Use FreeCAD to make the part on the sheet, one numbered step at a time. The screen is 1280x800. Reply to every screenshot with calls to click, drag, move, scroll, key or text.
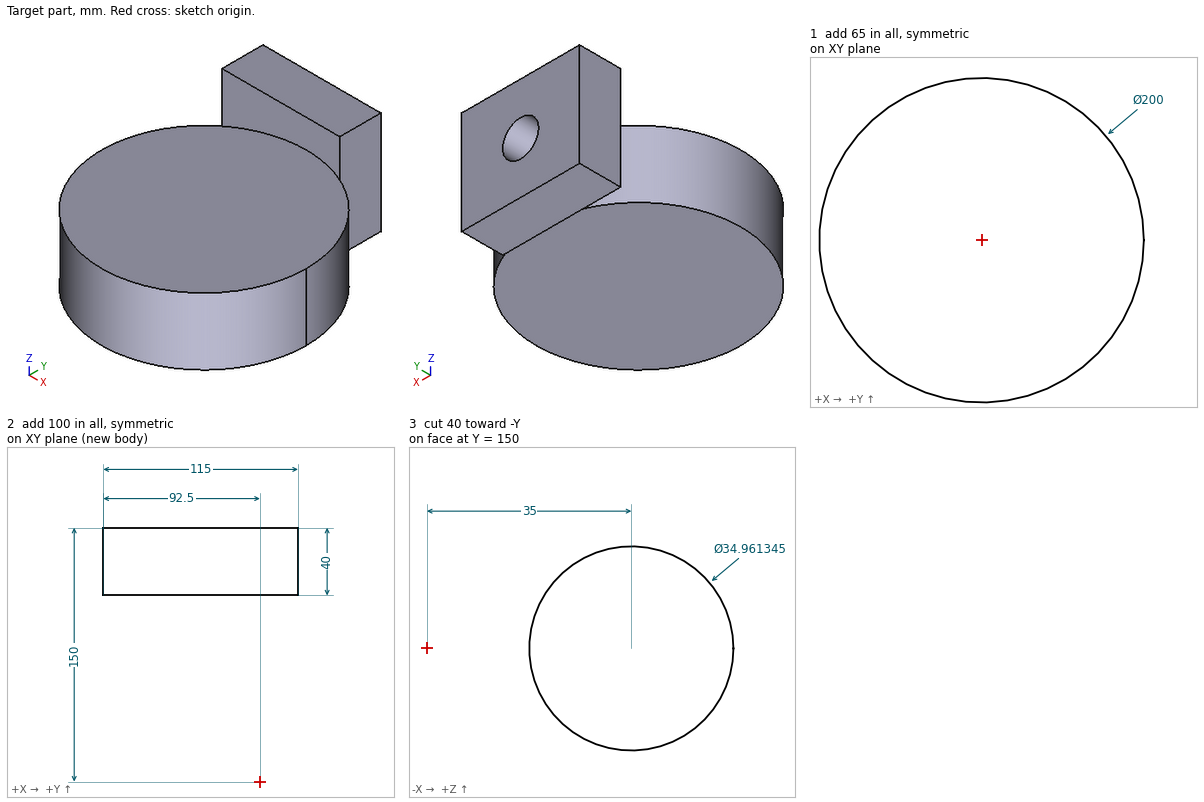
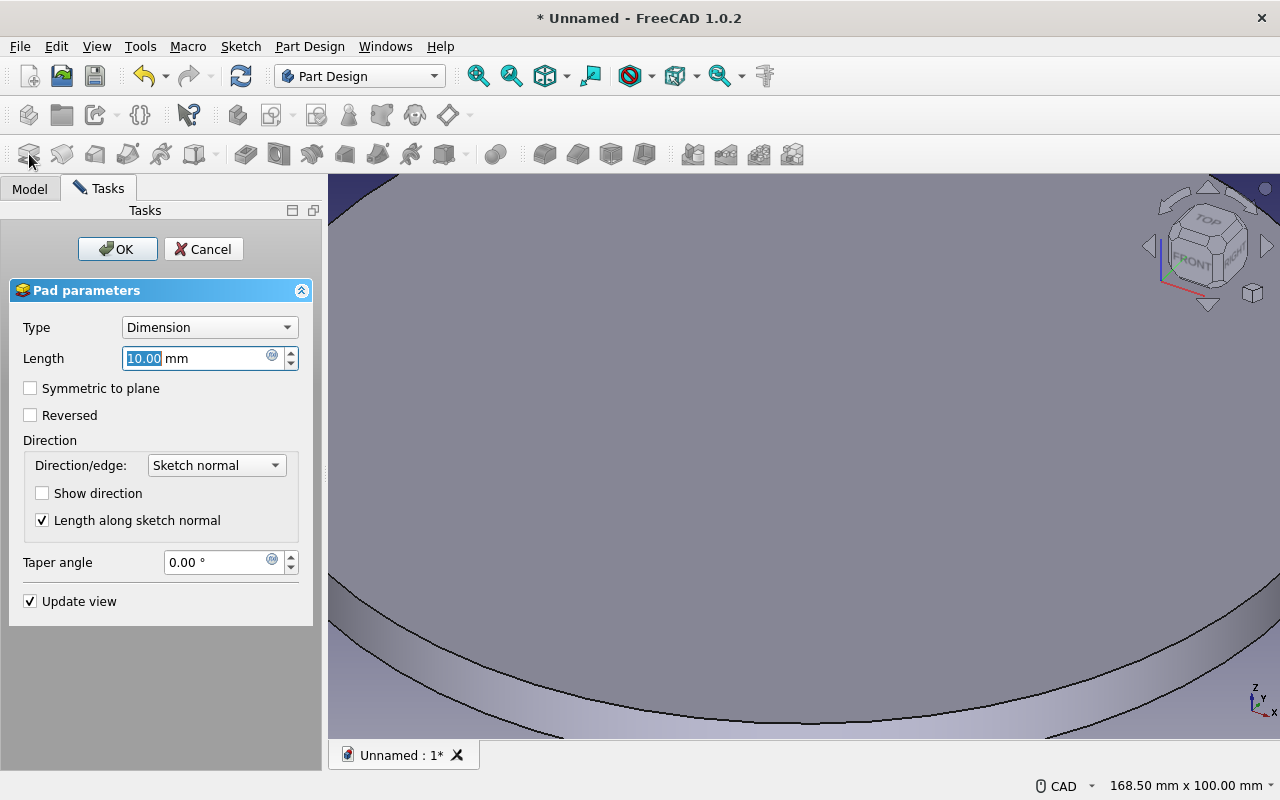
text(65)
key(Tab)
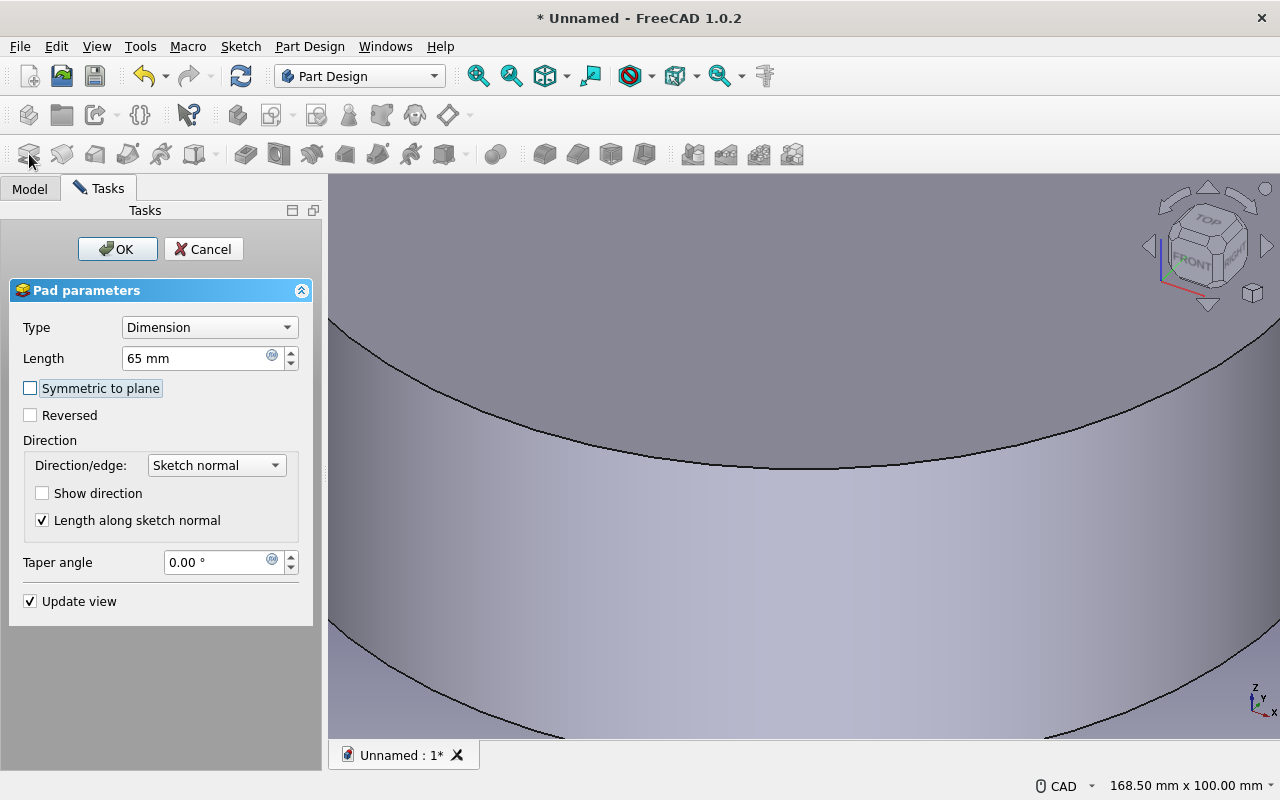
click(31, 388)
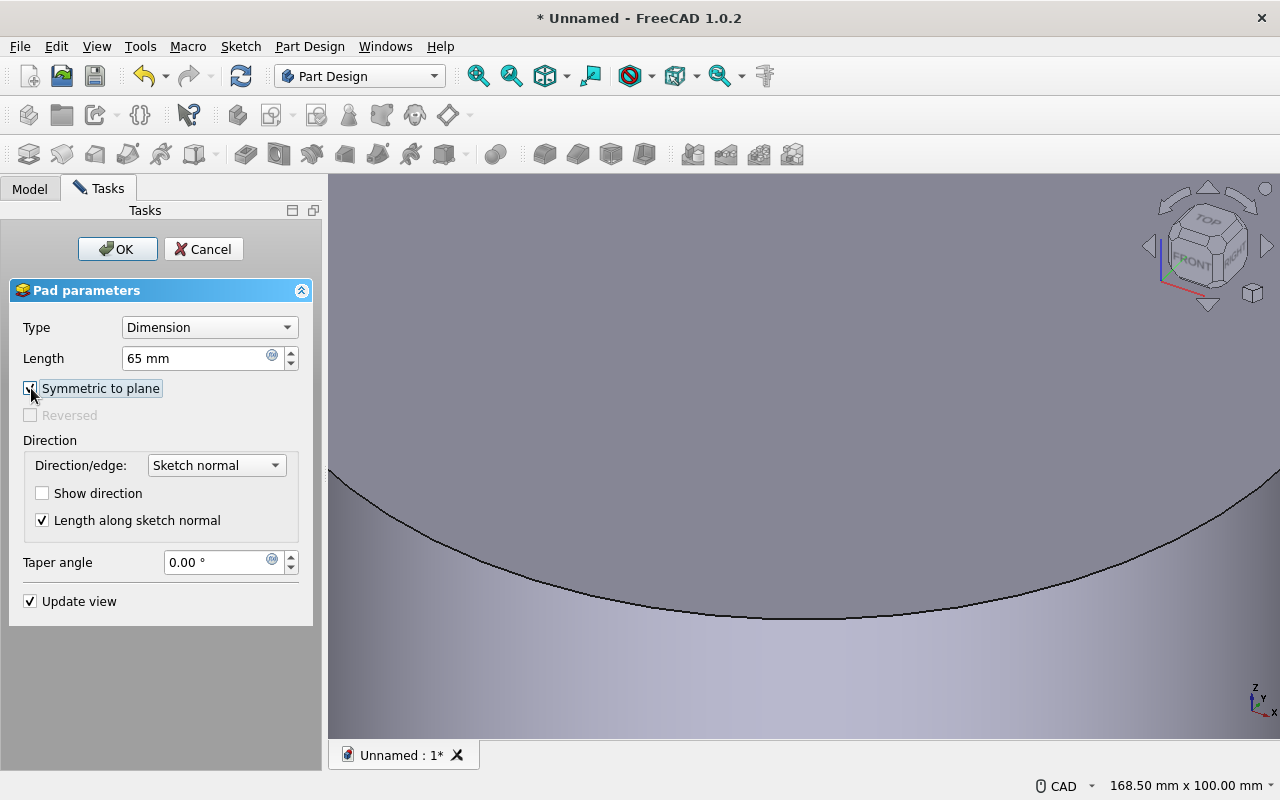
click(118, 249)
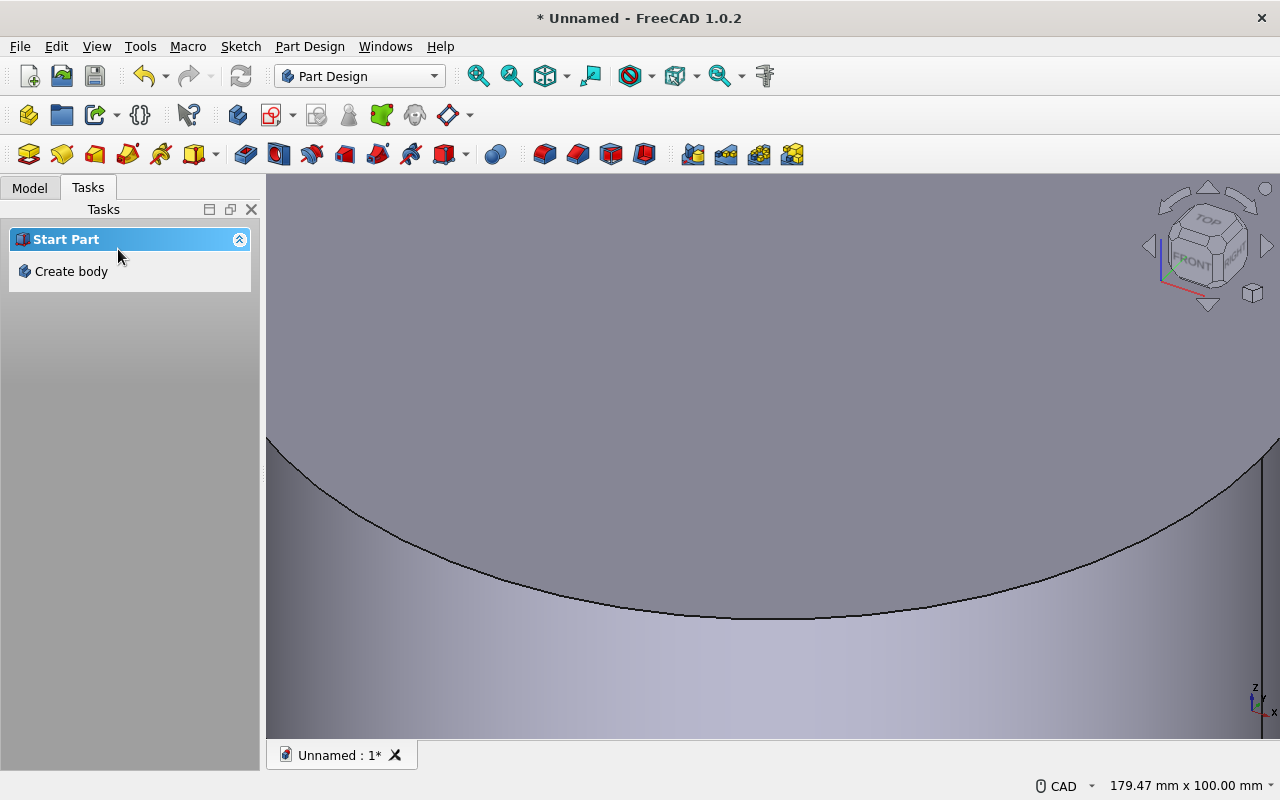
key(v)
key(f)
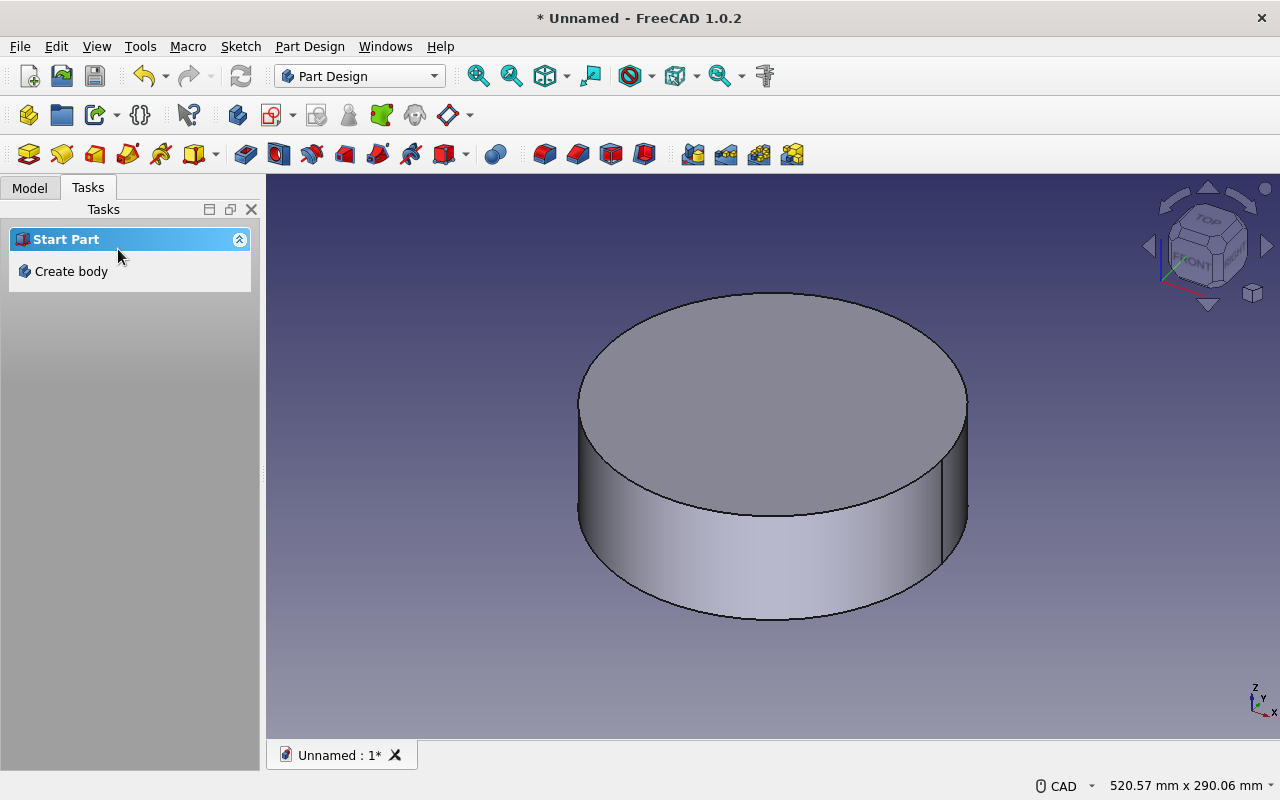
click(238, 116)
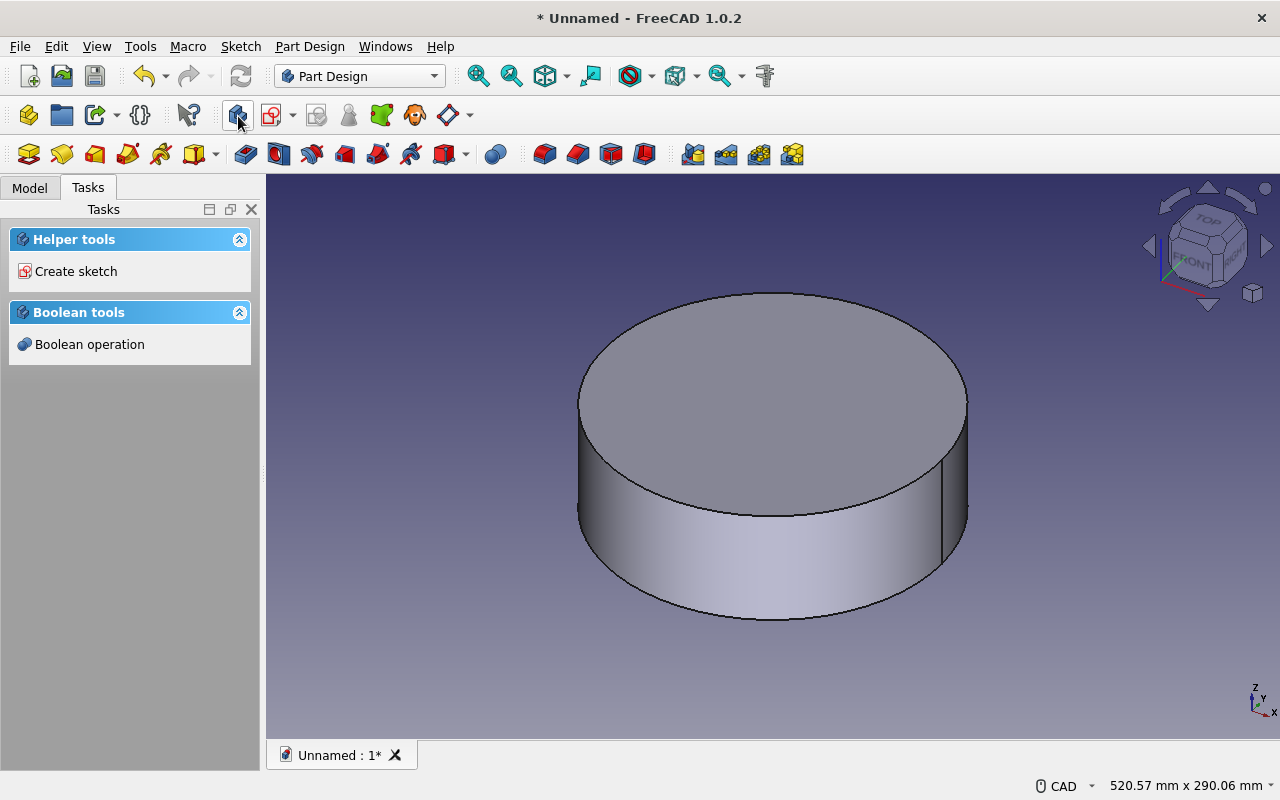
click(306, 699)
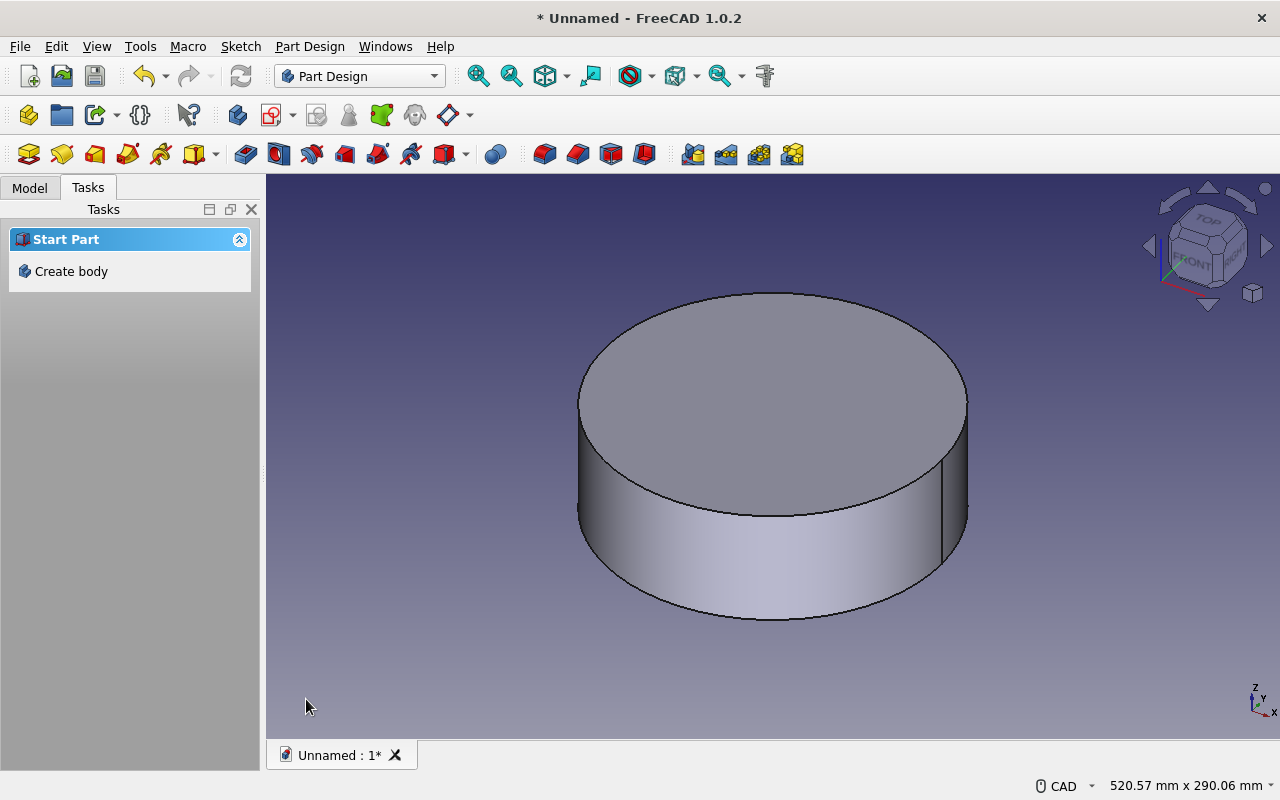
click(270, 116)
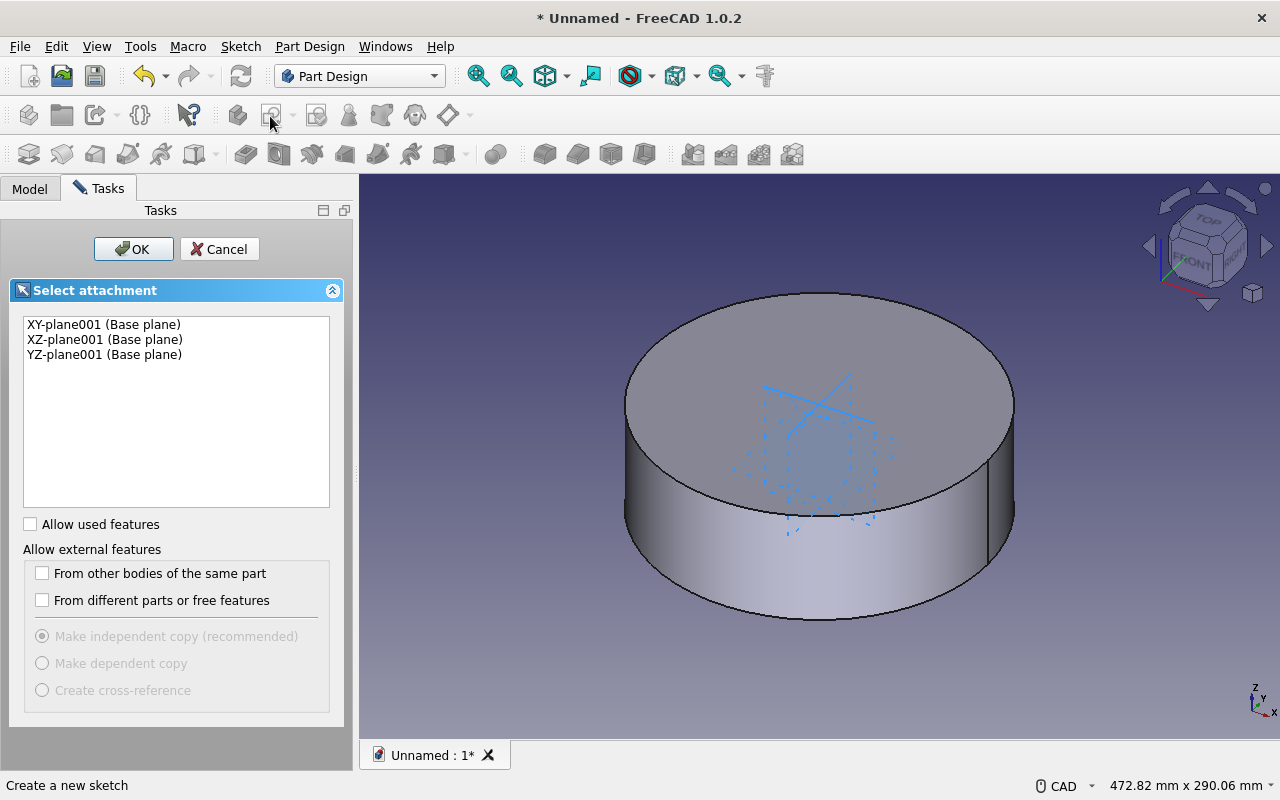
click(84, 324)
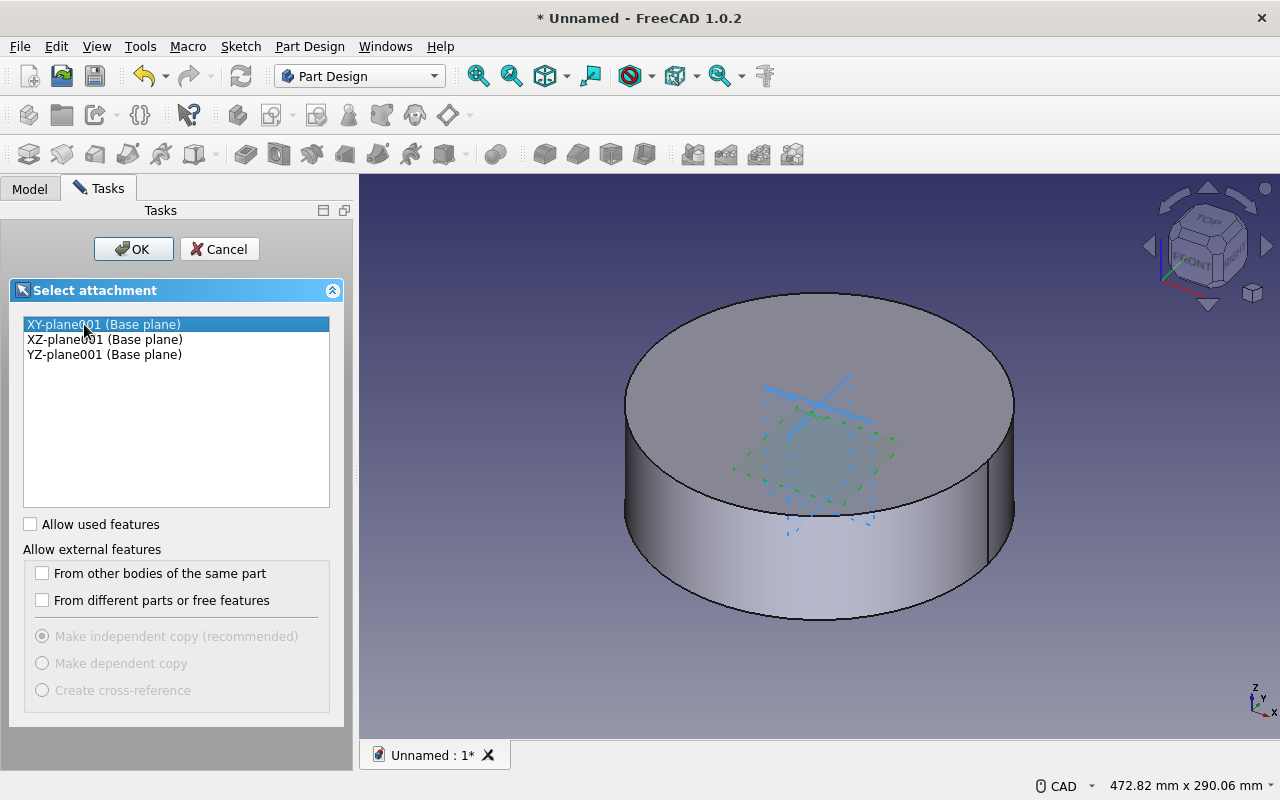
click(134, 249)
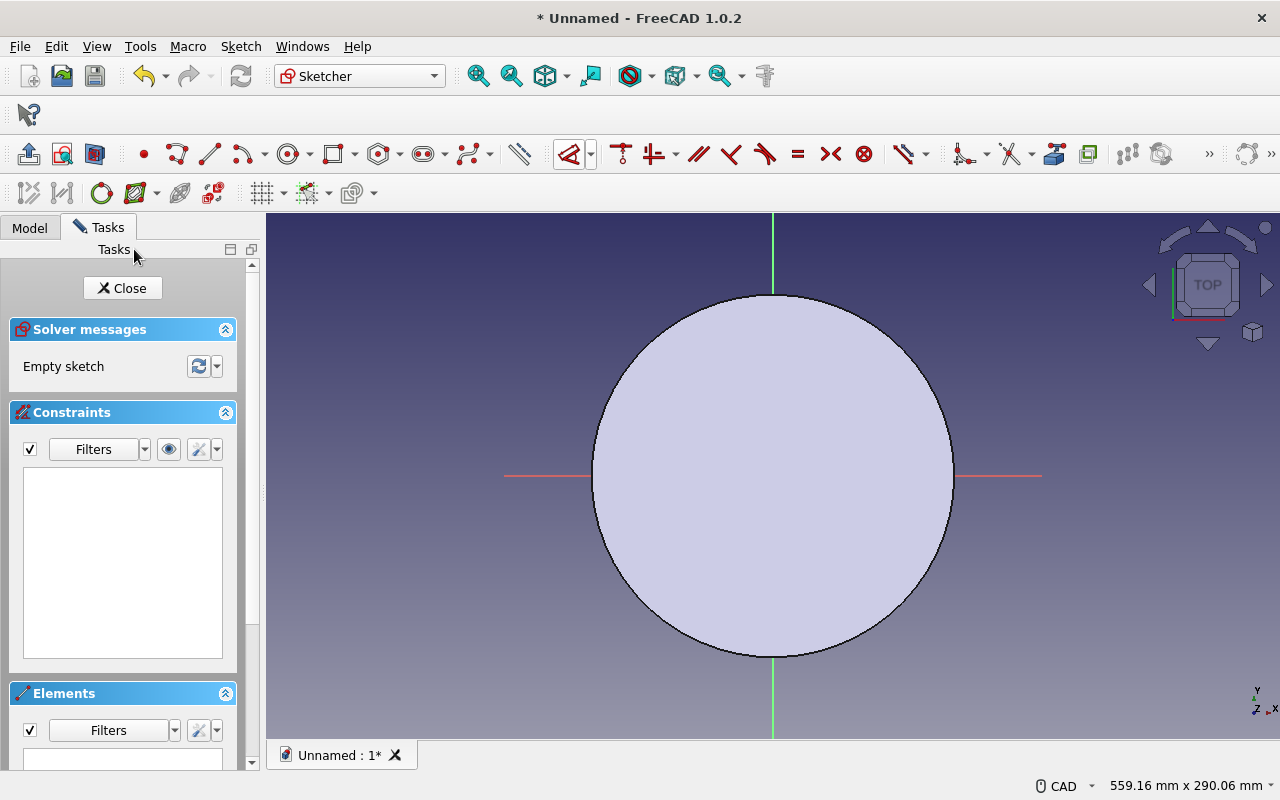
scroll(682, 711, down, 1)